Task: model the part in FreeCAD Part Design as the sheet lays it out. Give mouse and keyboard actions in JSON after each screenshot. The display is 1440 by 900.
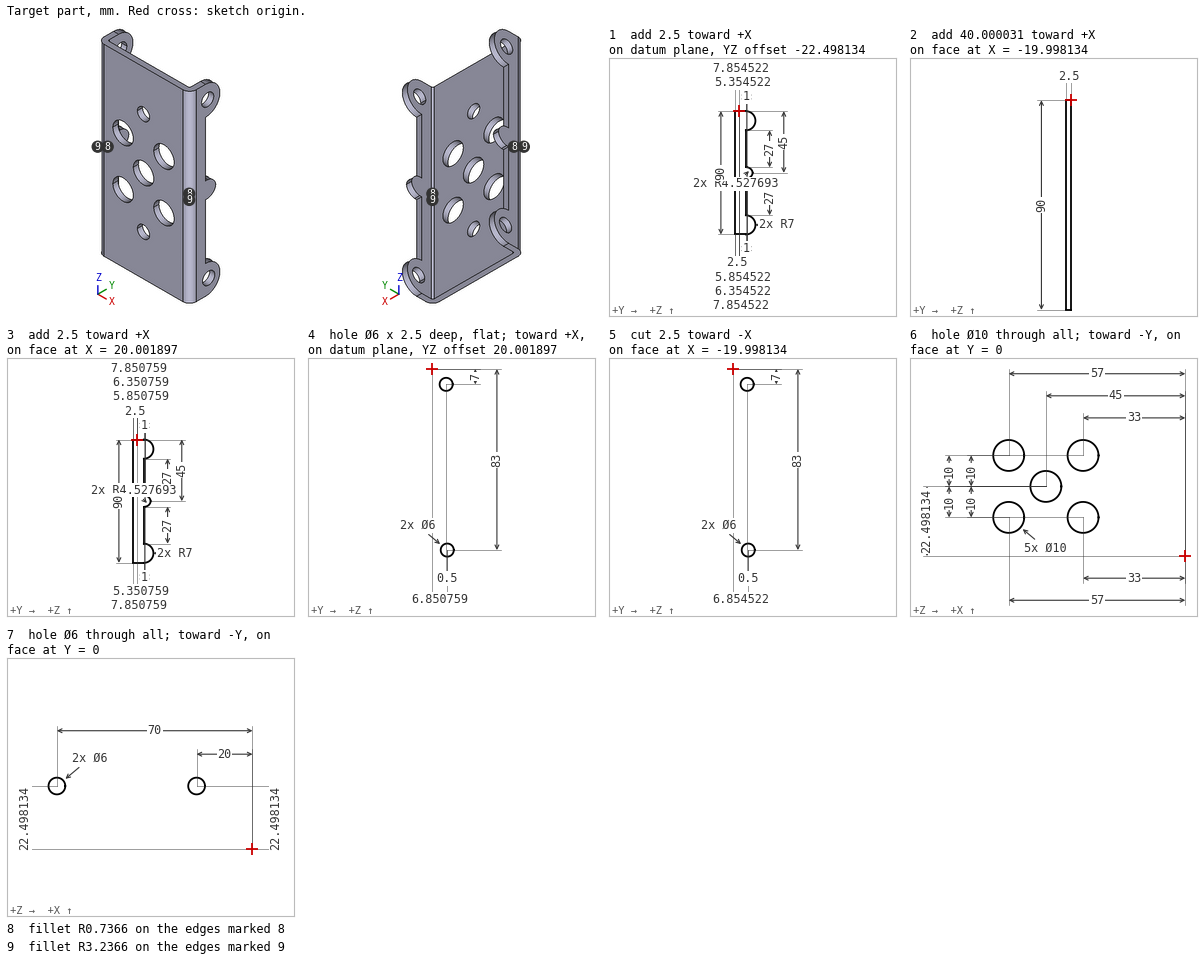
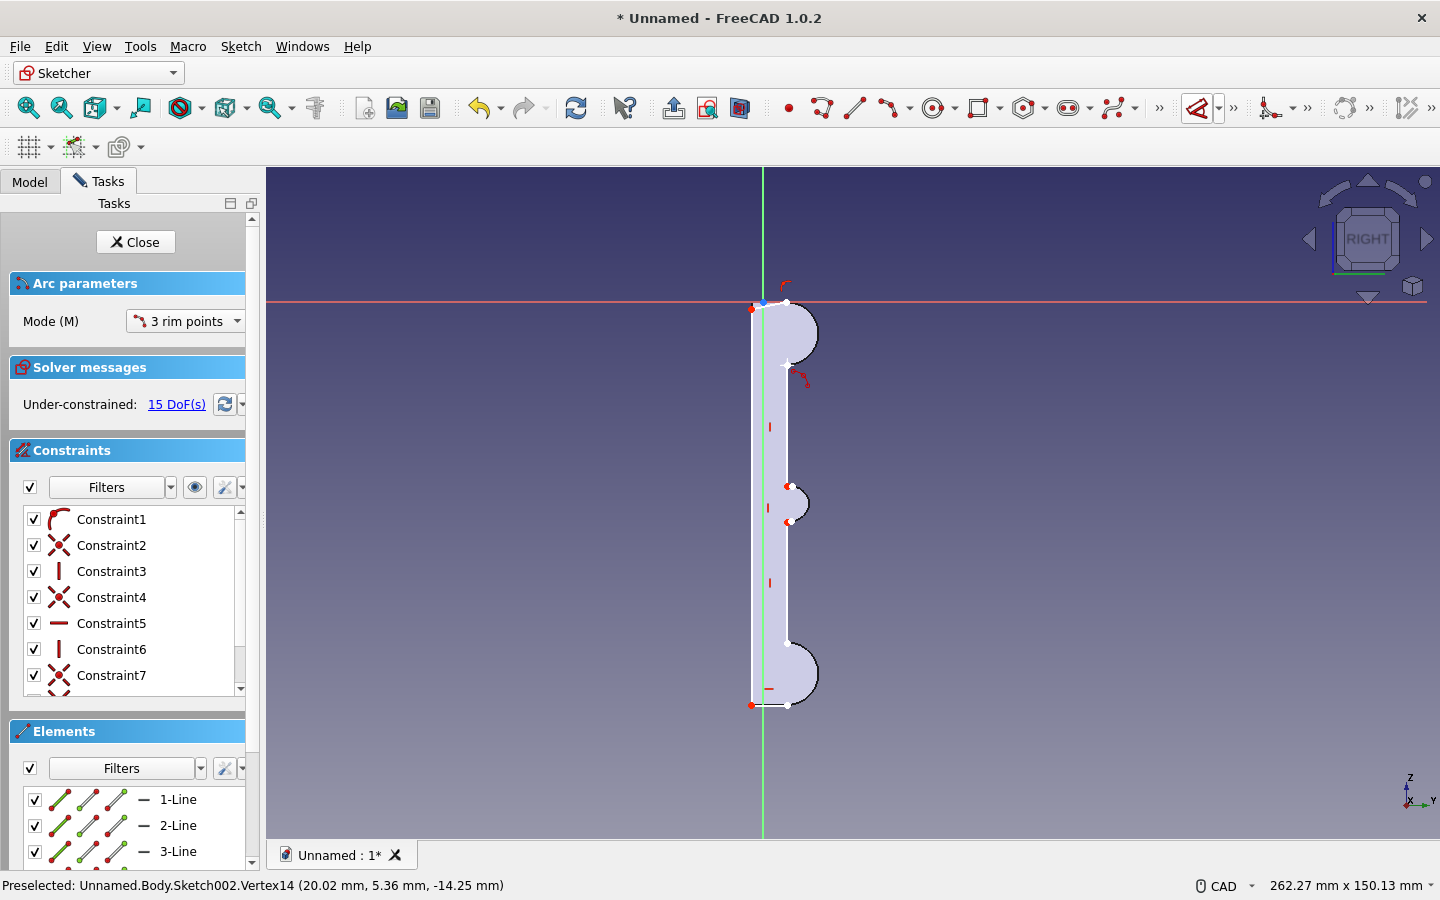
{"action": "left_click", "coordinate": [787, 706]}
{"action": "left_click", "coordinate": [787, 643]}
{"action": "left_click", "coordinate": [818, 674]}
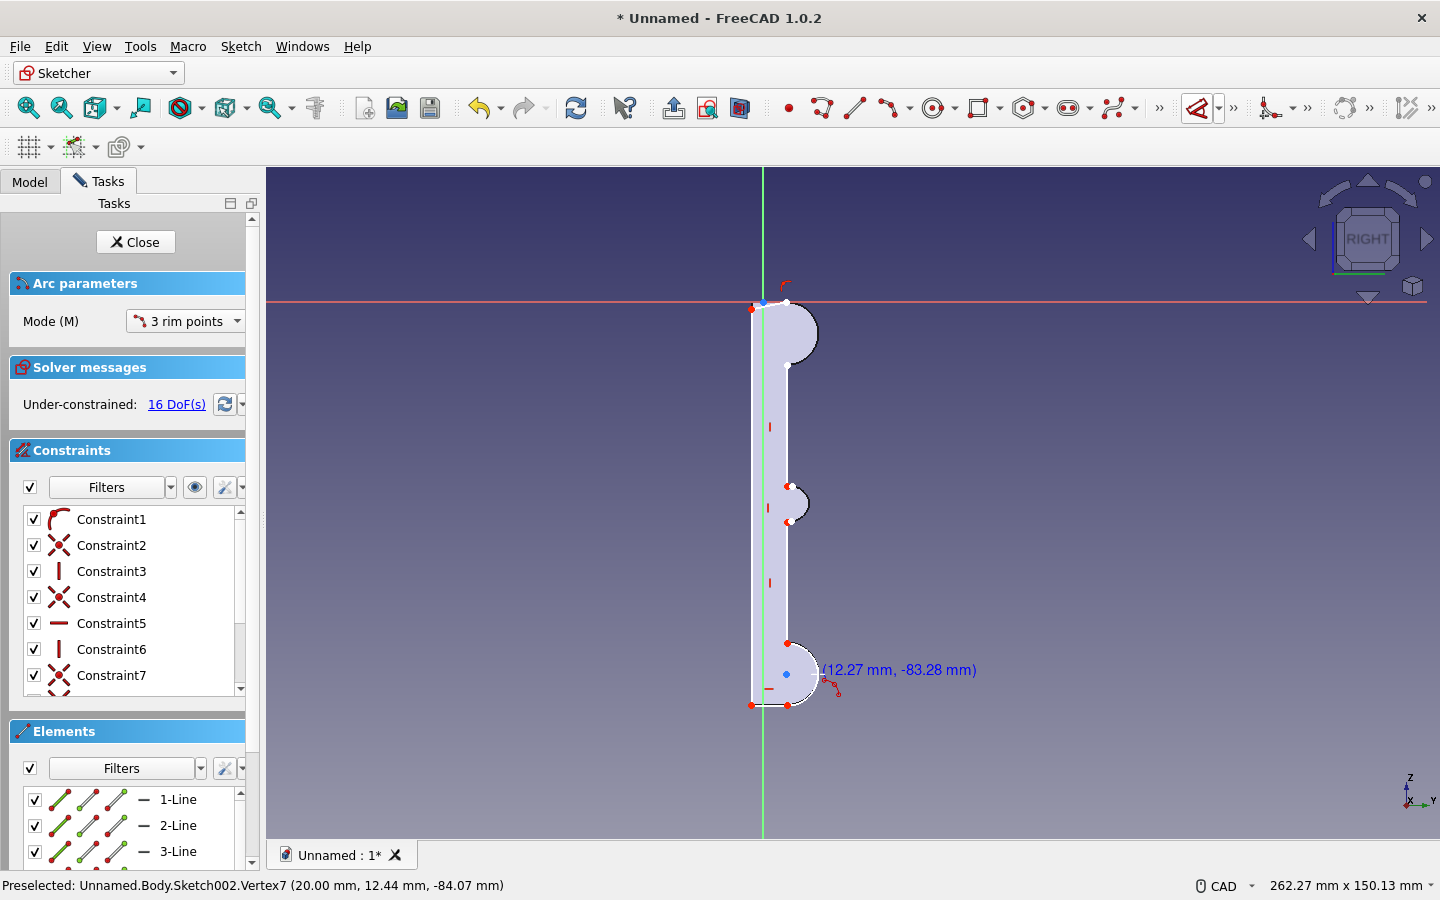
{"action": "scroll", "coordinate": [792, 522], "scroll_direction": "up", "scroll_amount": 10}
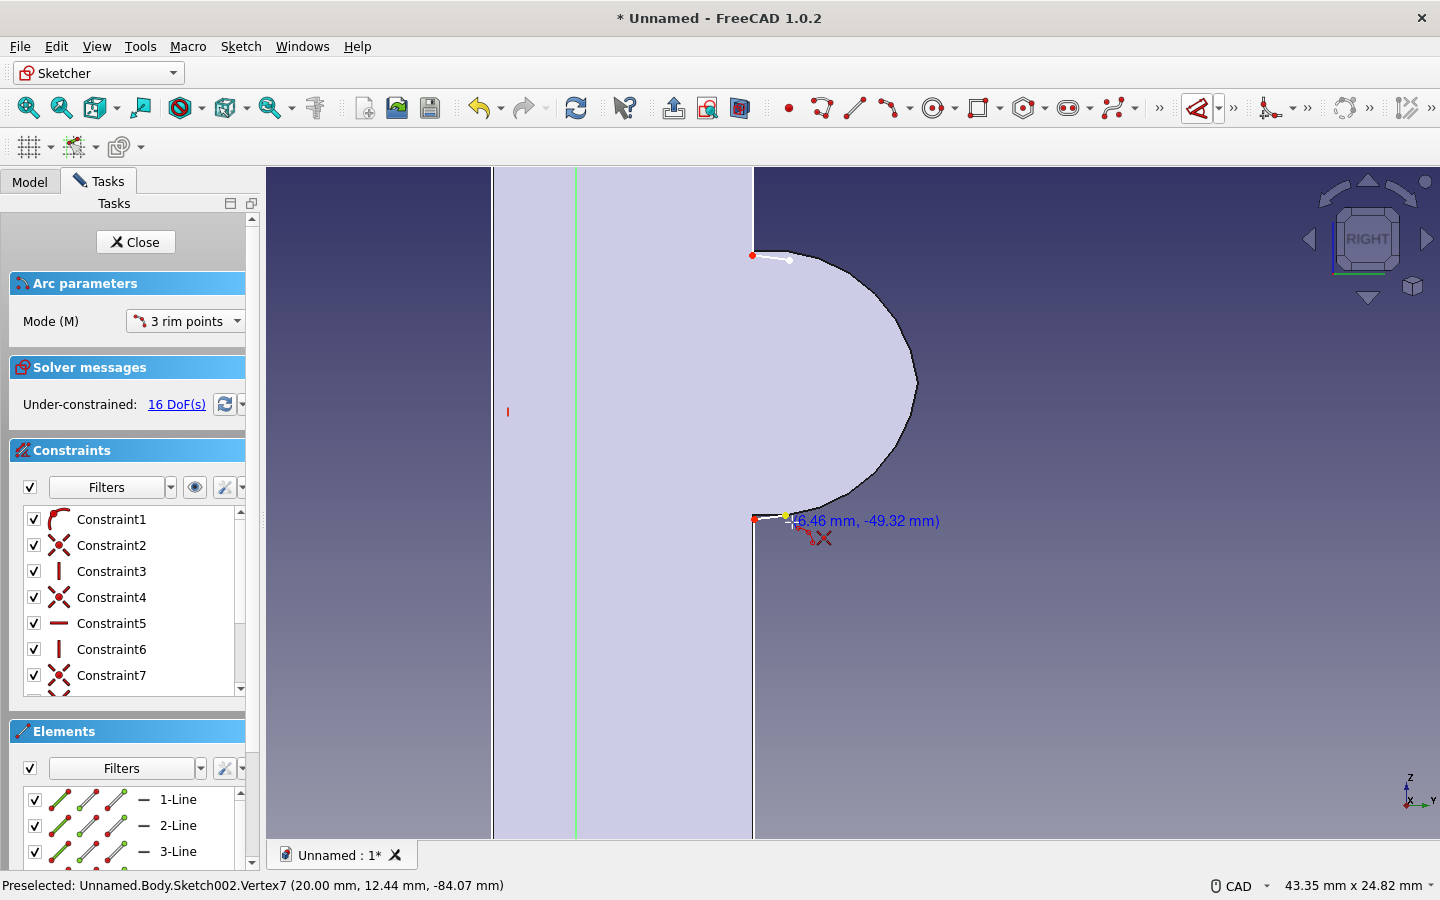
{"action": "left_click", "coordinate": [785, 516]}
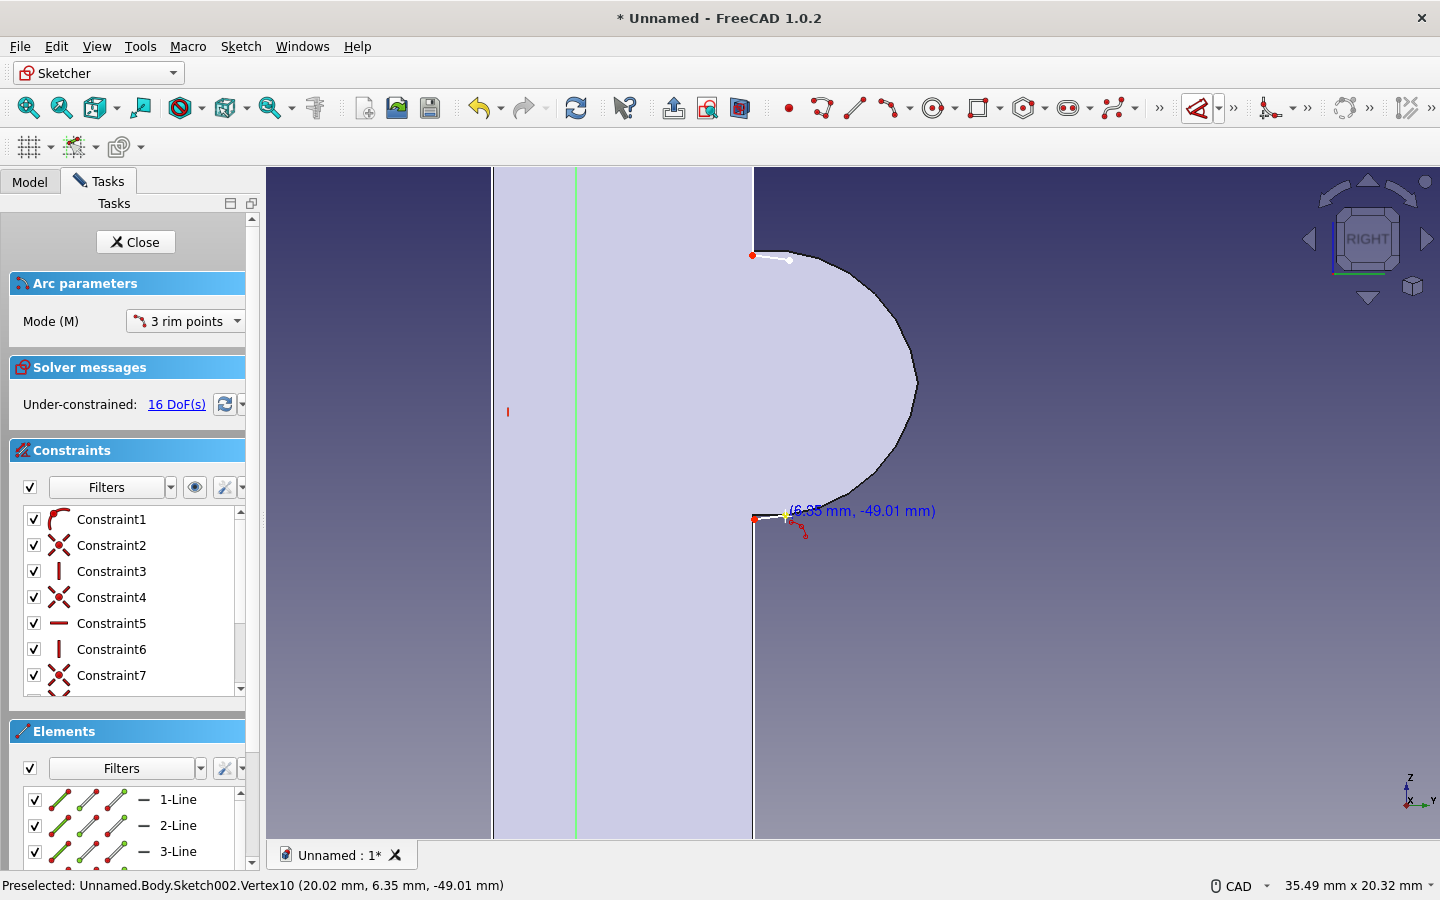
{"action": "scroll", "coordinate": [792, 522], "scroll_direction": "down", "scroll_amount": 10}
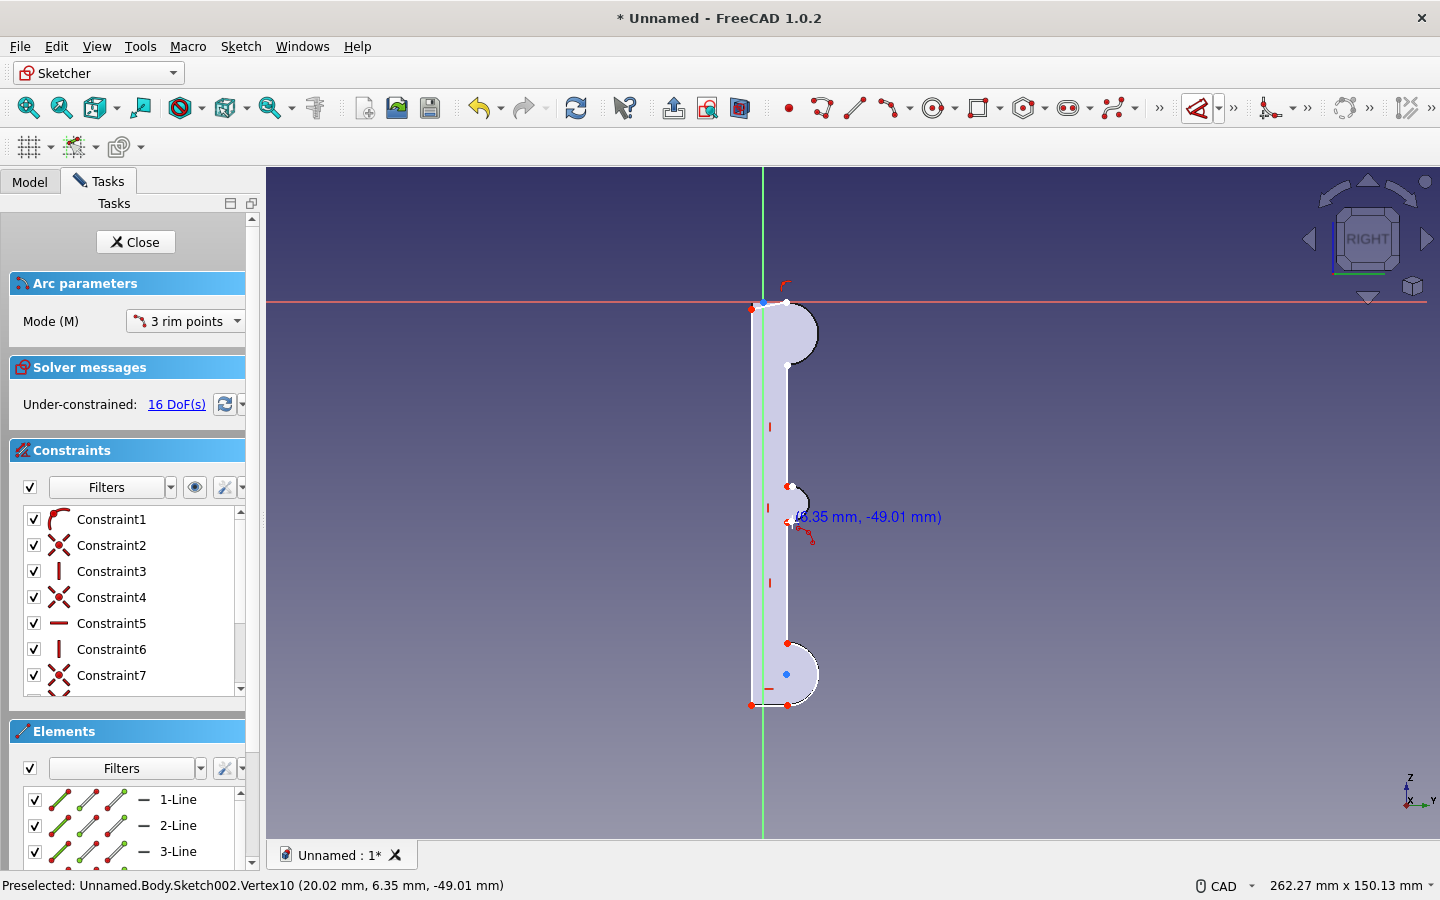
{"action": "left_click", "coordinate": [809, 504]}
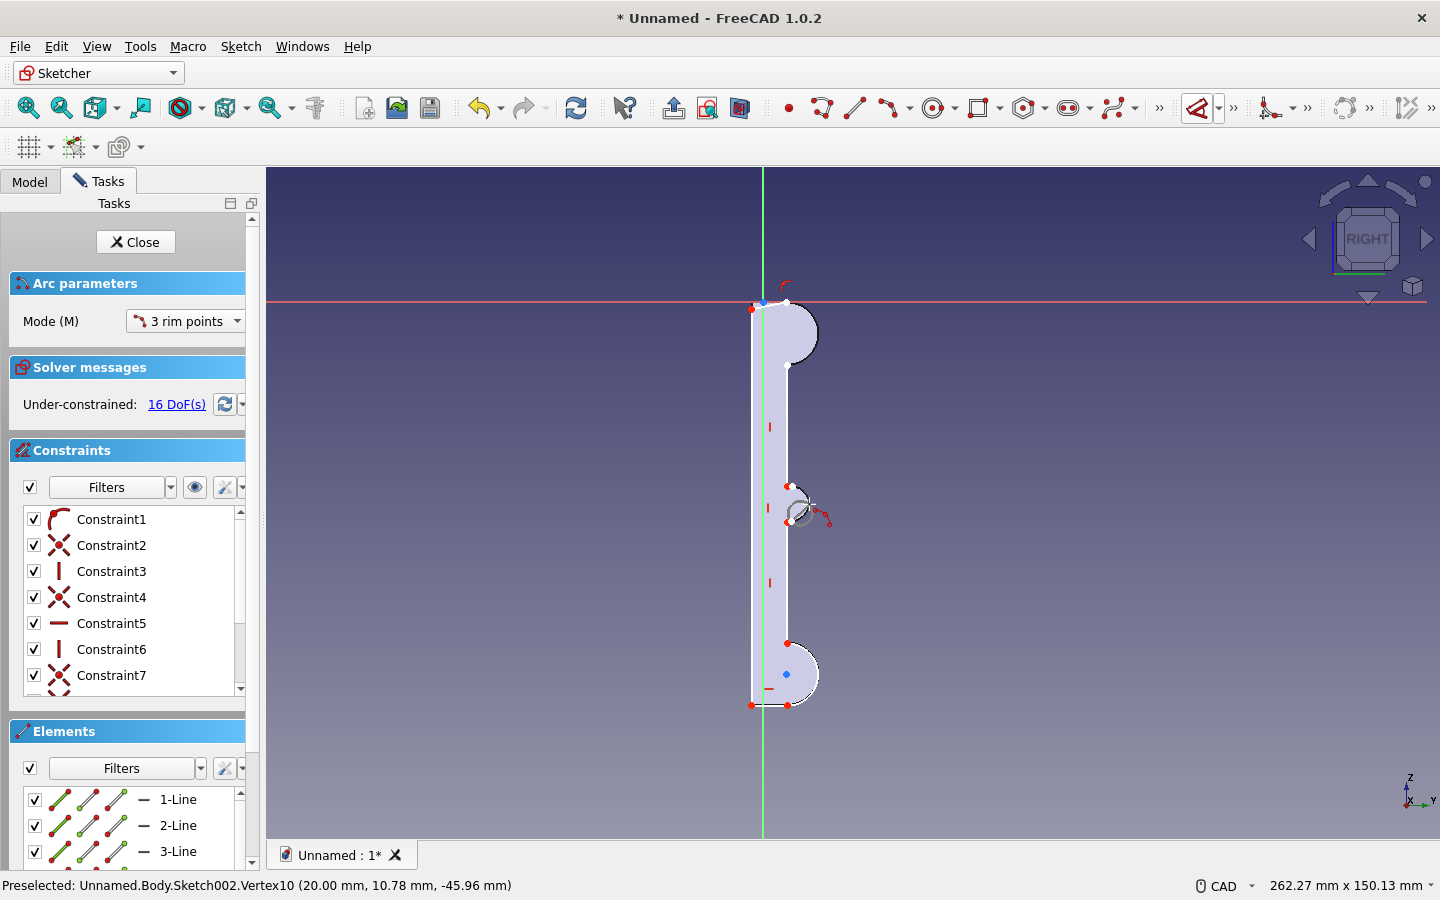
{"action": "scroll", "coordinate": [804, 516], "scroll_direction": "up", "scroll_amount": 7}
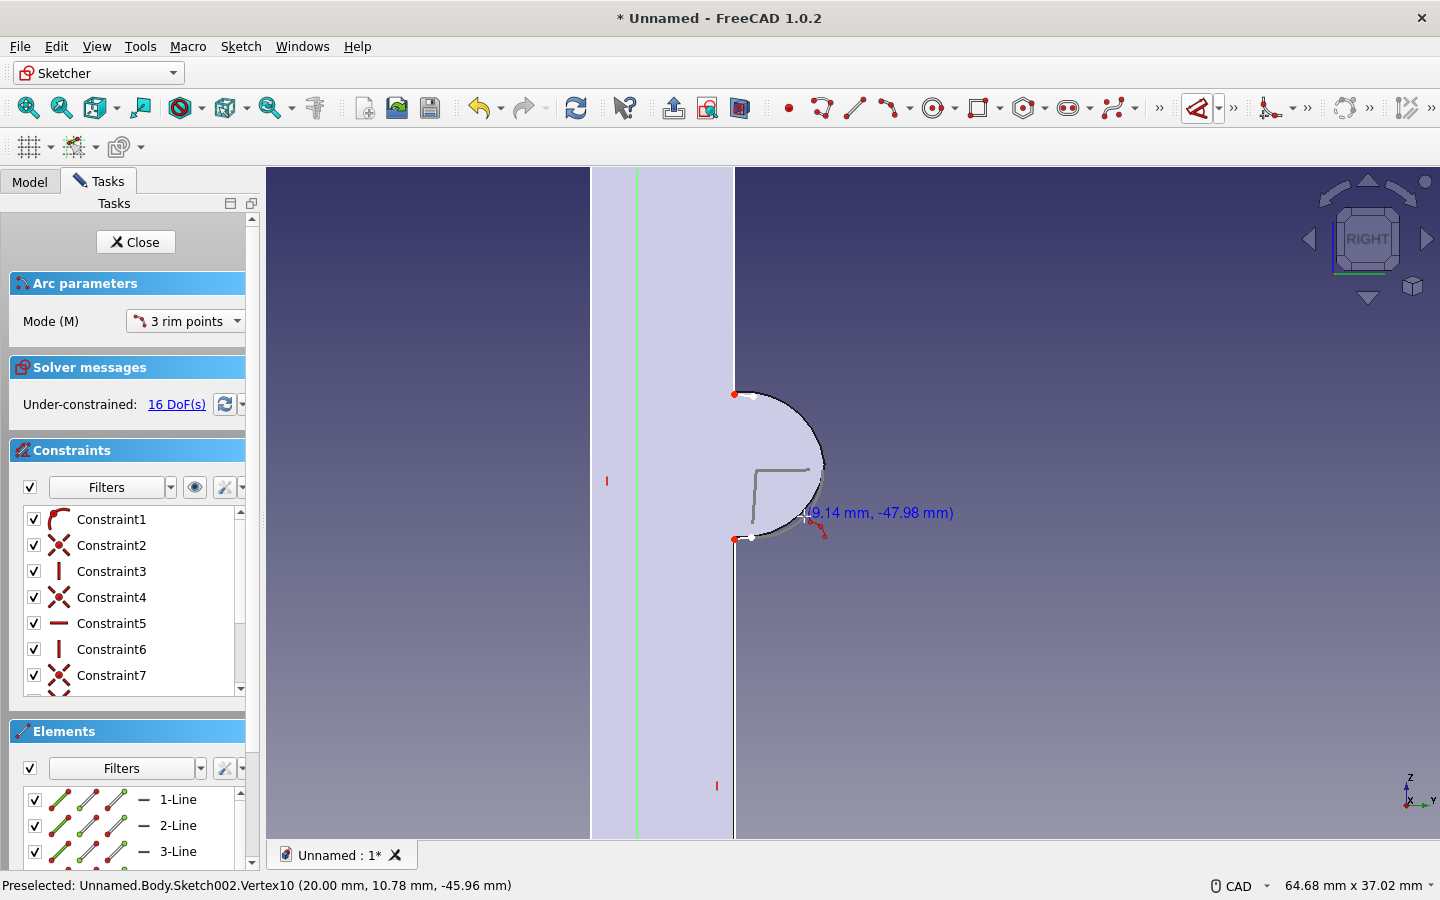
{"action": "left_click", "coordinate": [801, 513]}